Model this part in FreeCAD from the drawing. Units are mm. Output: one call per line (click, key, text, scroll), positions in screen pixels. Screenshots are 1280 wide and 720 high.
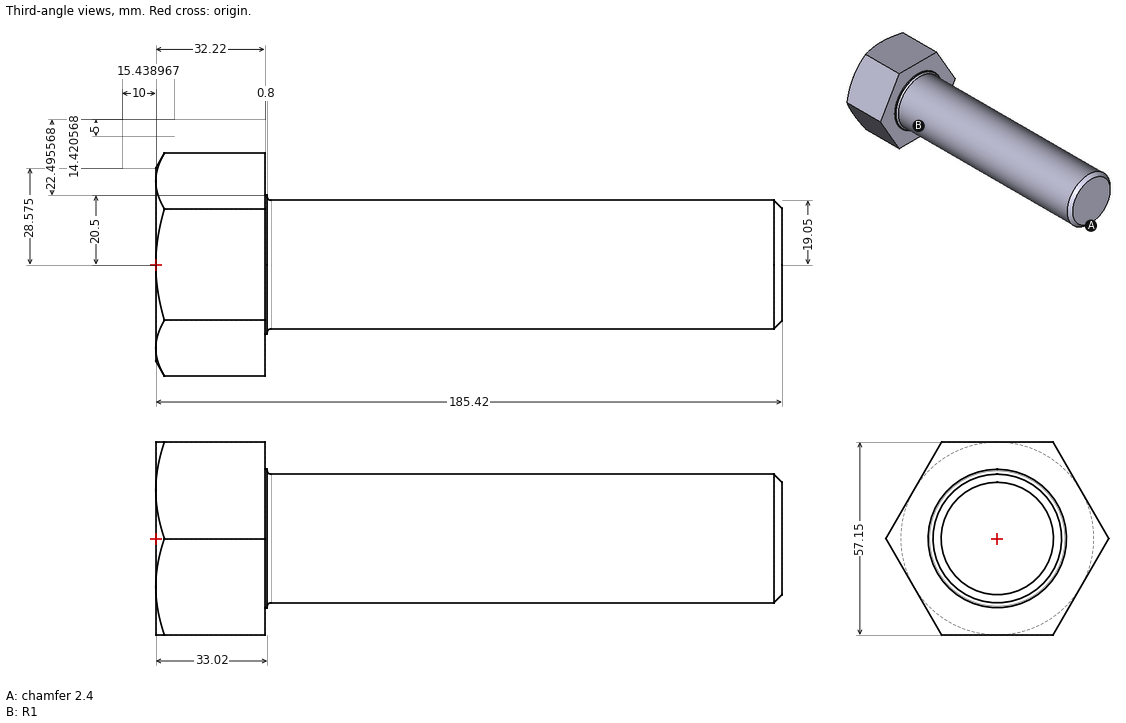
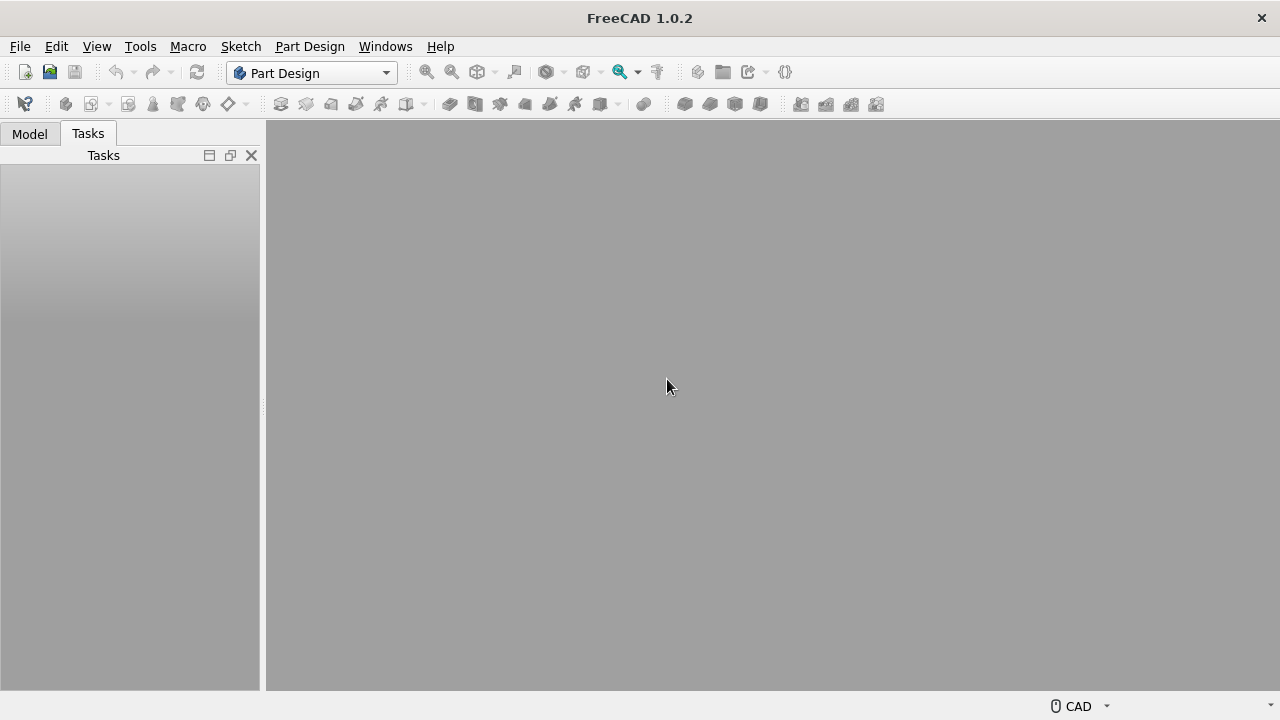
click(25, 72)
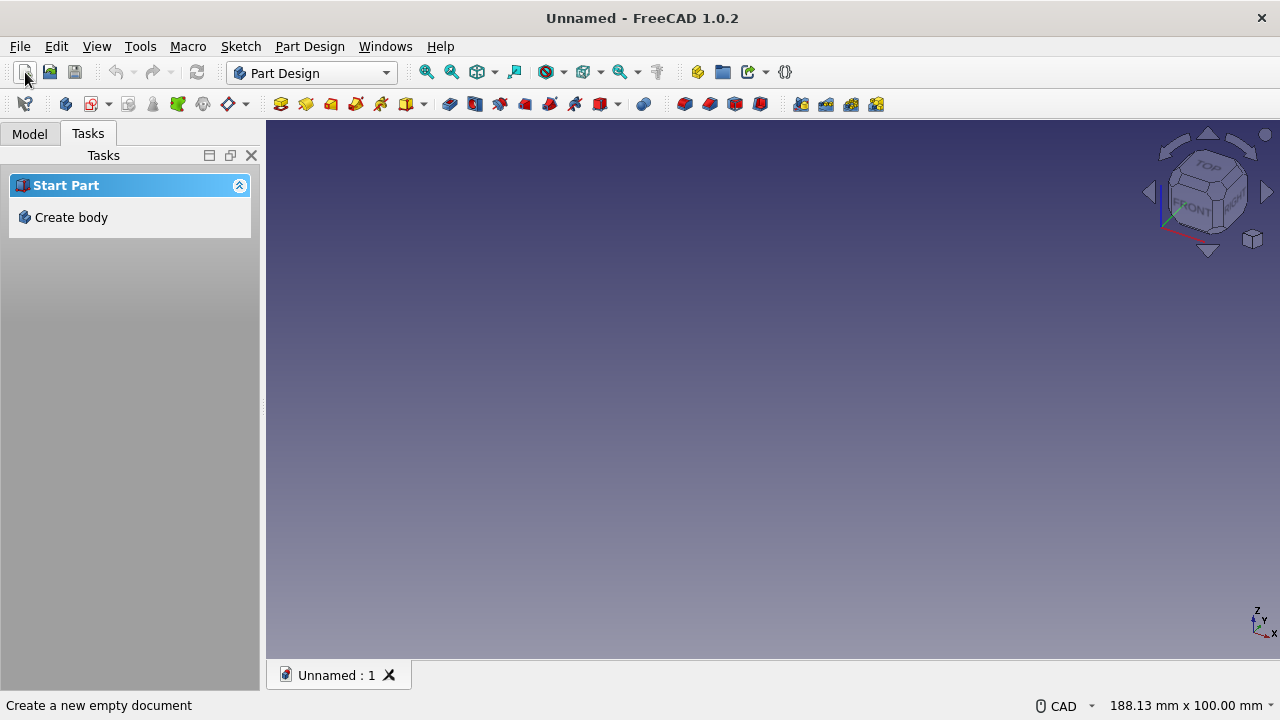
click(90, 104)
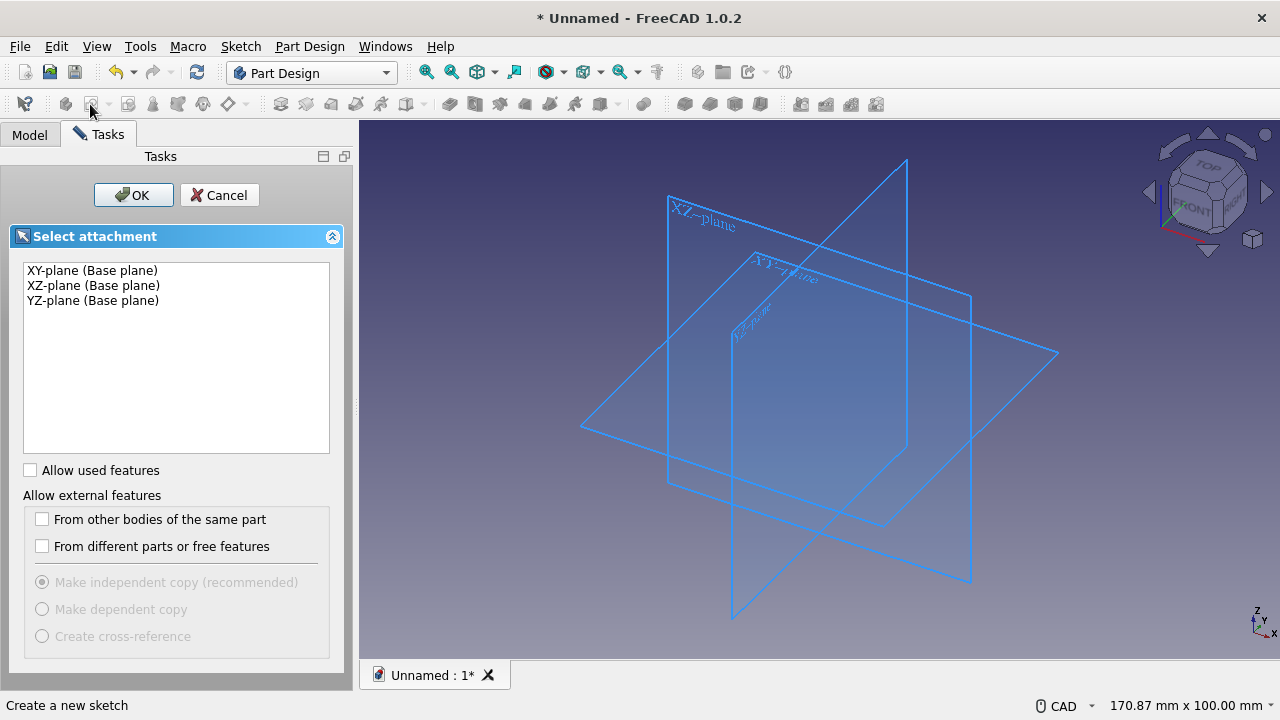
click(84, 300)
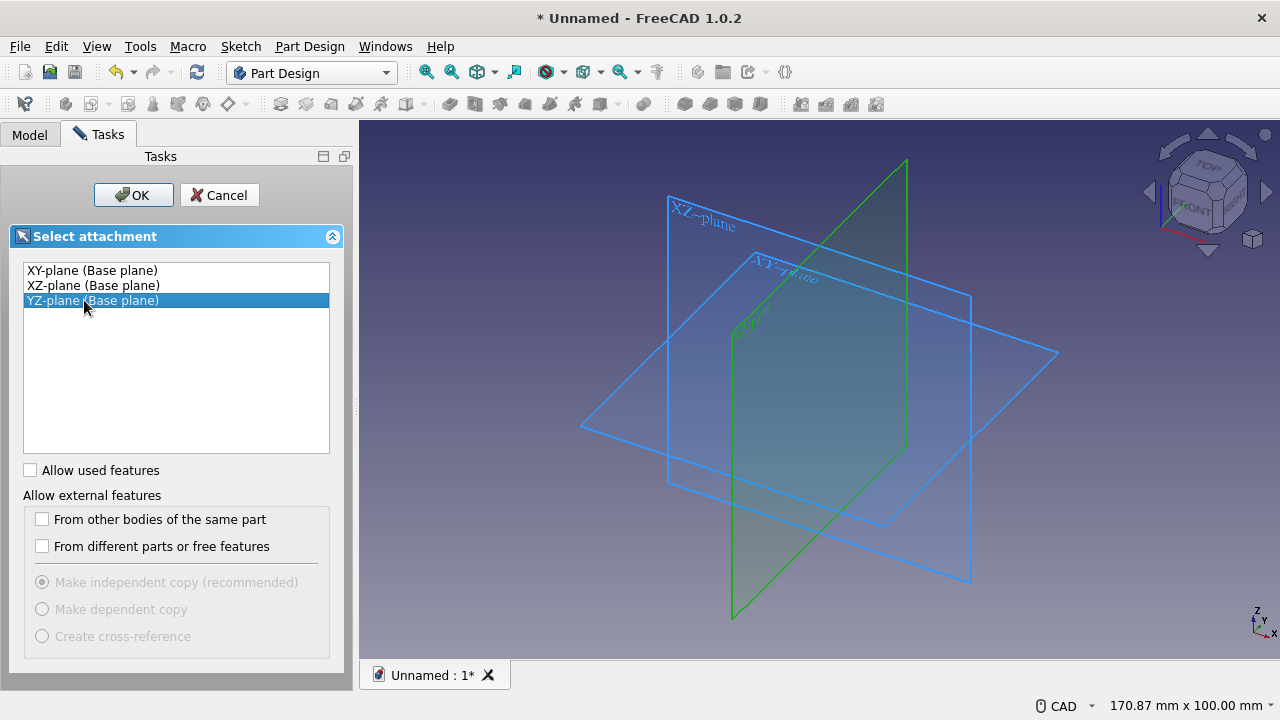
click(134, 195)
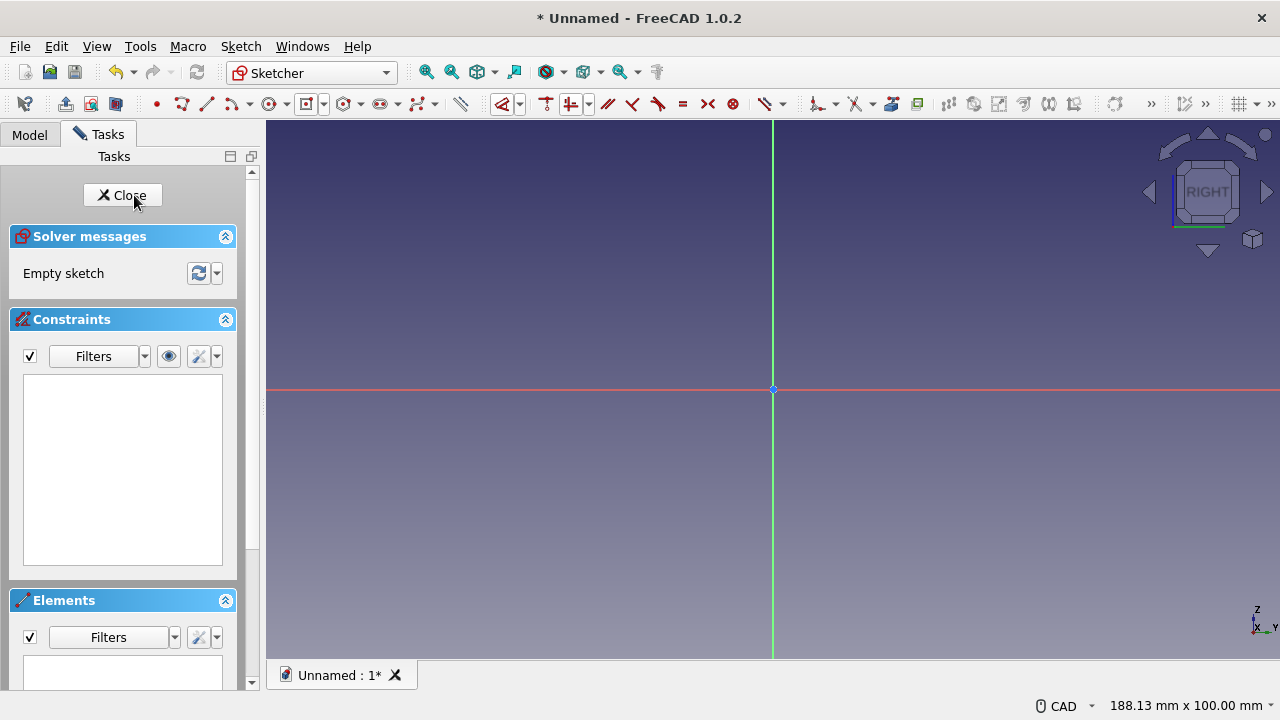
click(342, 104)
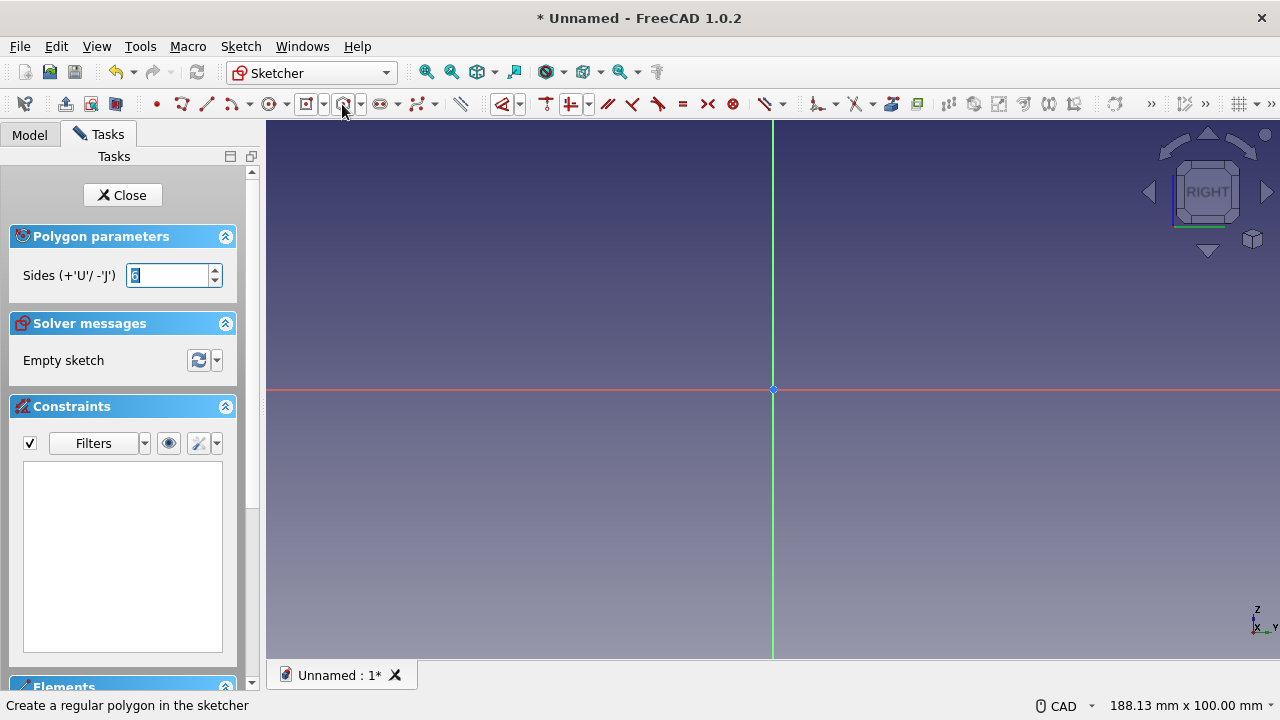
click(773, 390)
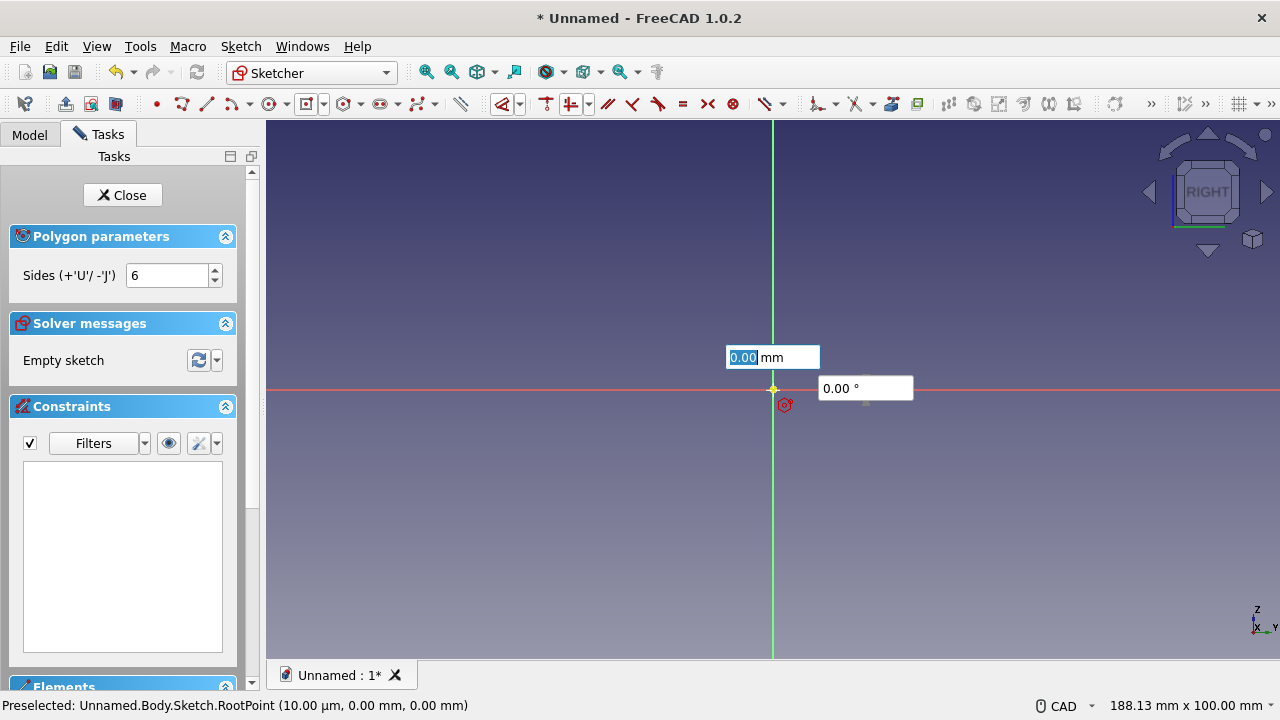
click(951, 390)
key(Escape)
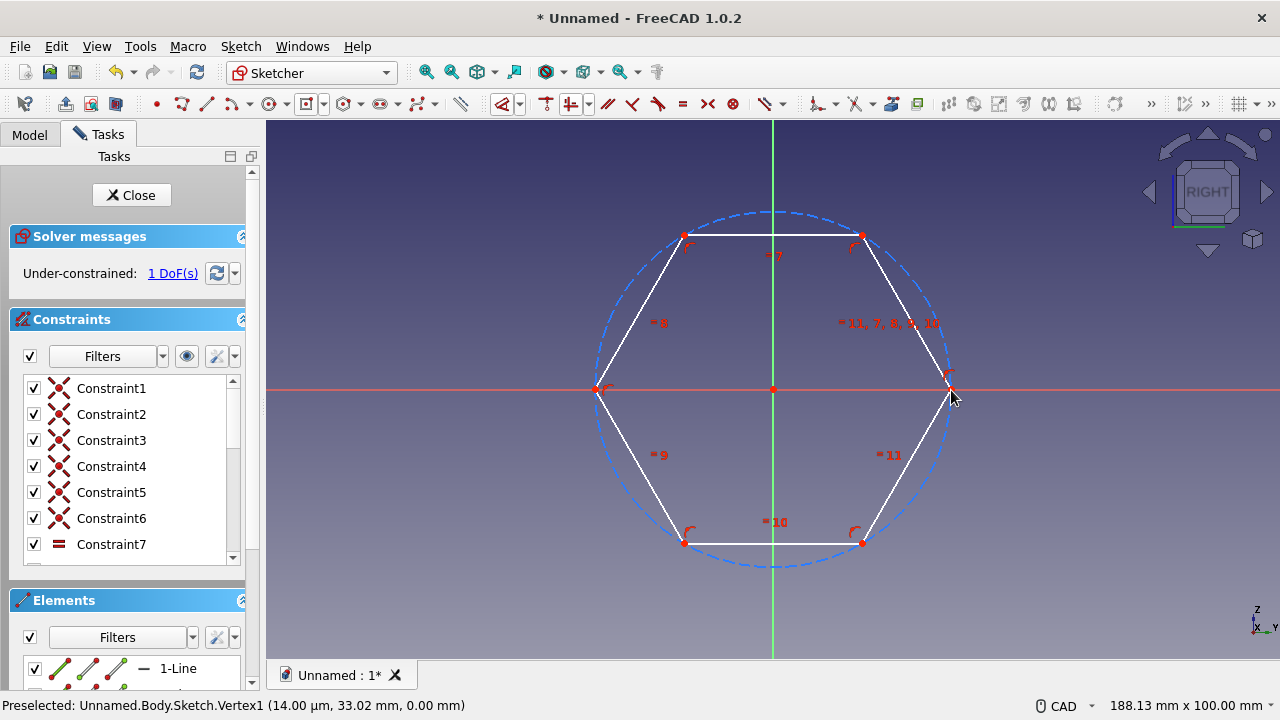
click(684, 544)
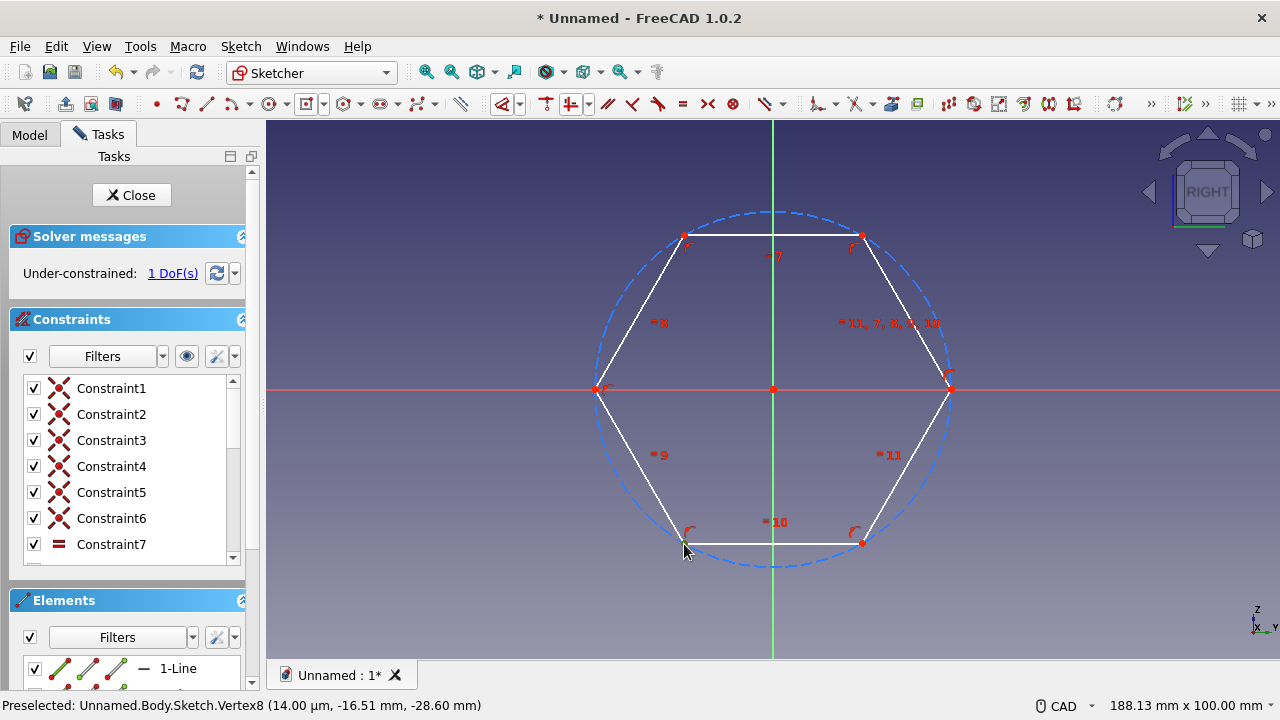
click(862, 235)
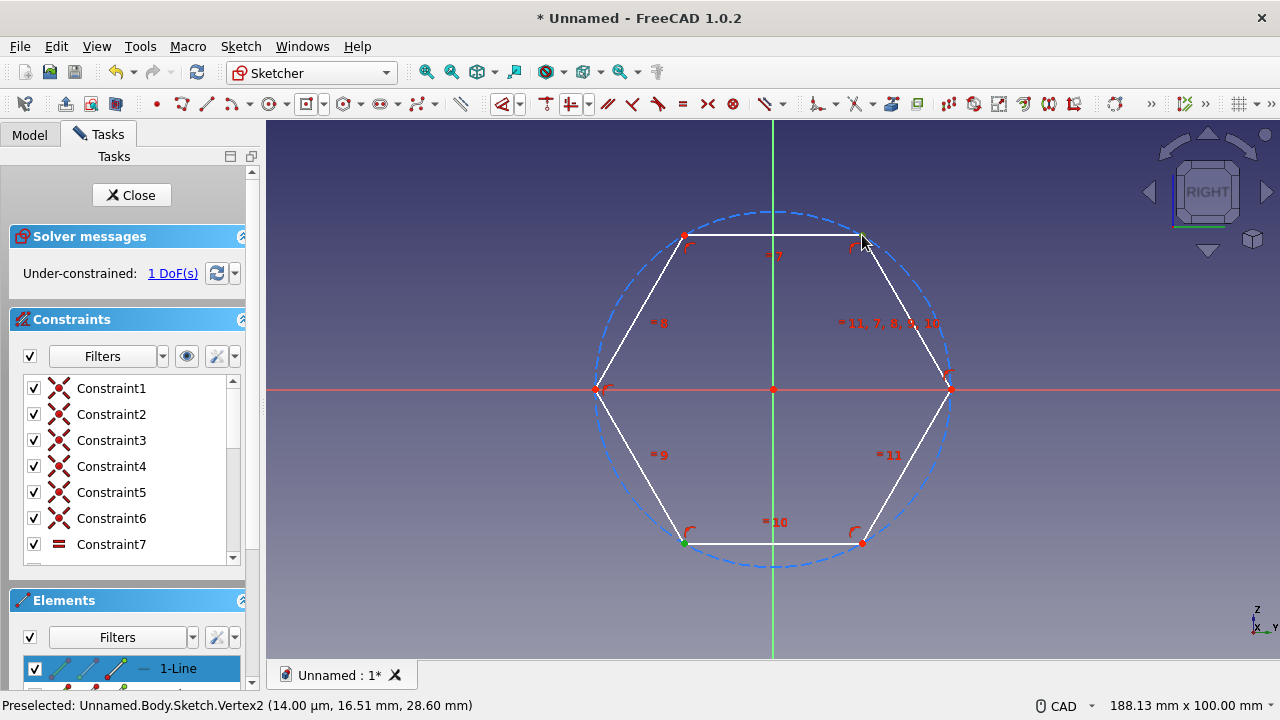
key(i)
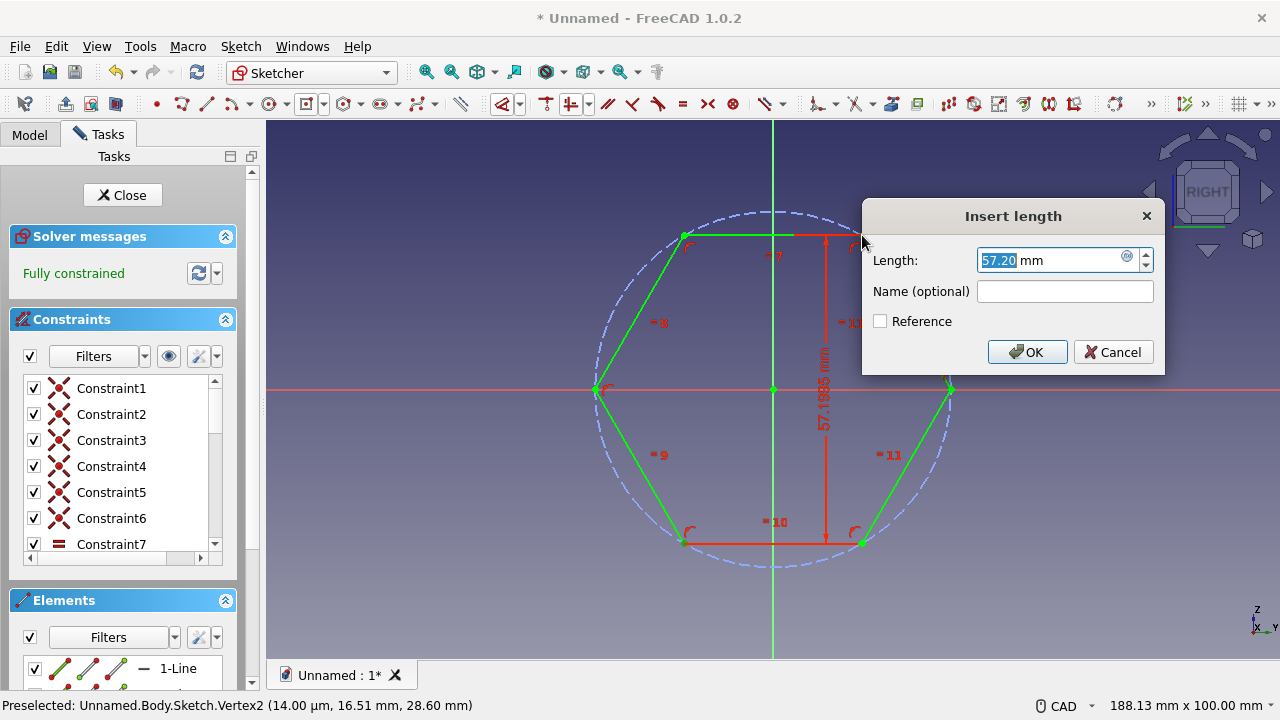
text(57.15)
key(Return)